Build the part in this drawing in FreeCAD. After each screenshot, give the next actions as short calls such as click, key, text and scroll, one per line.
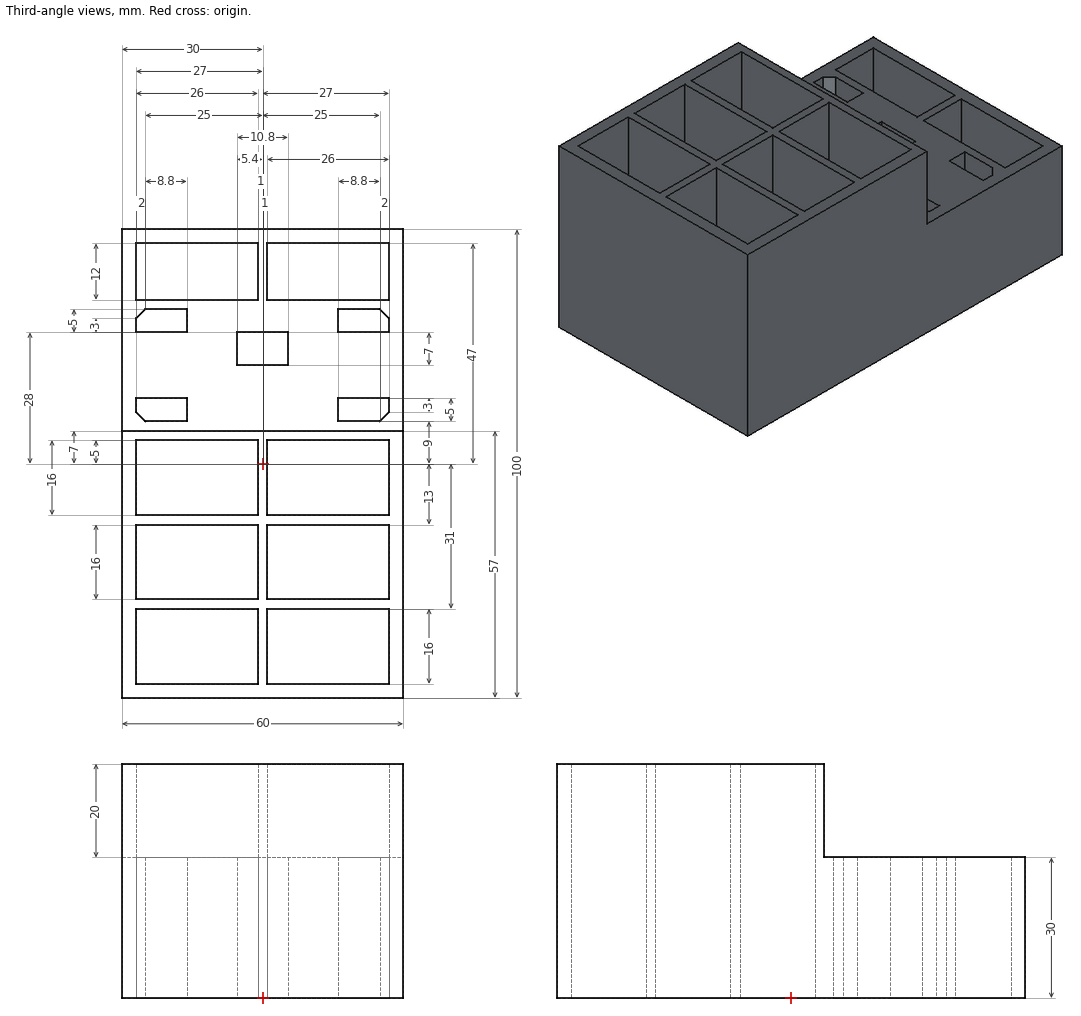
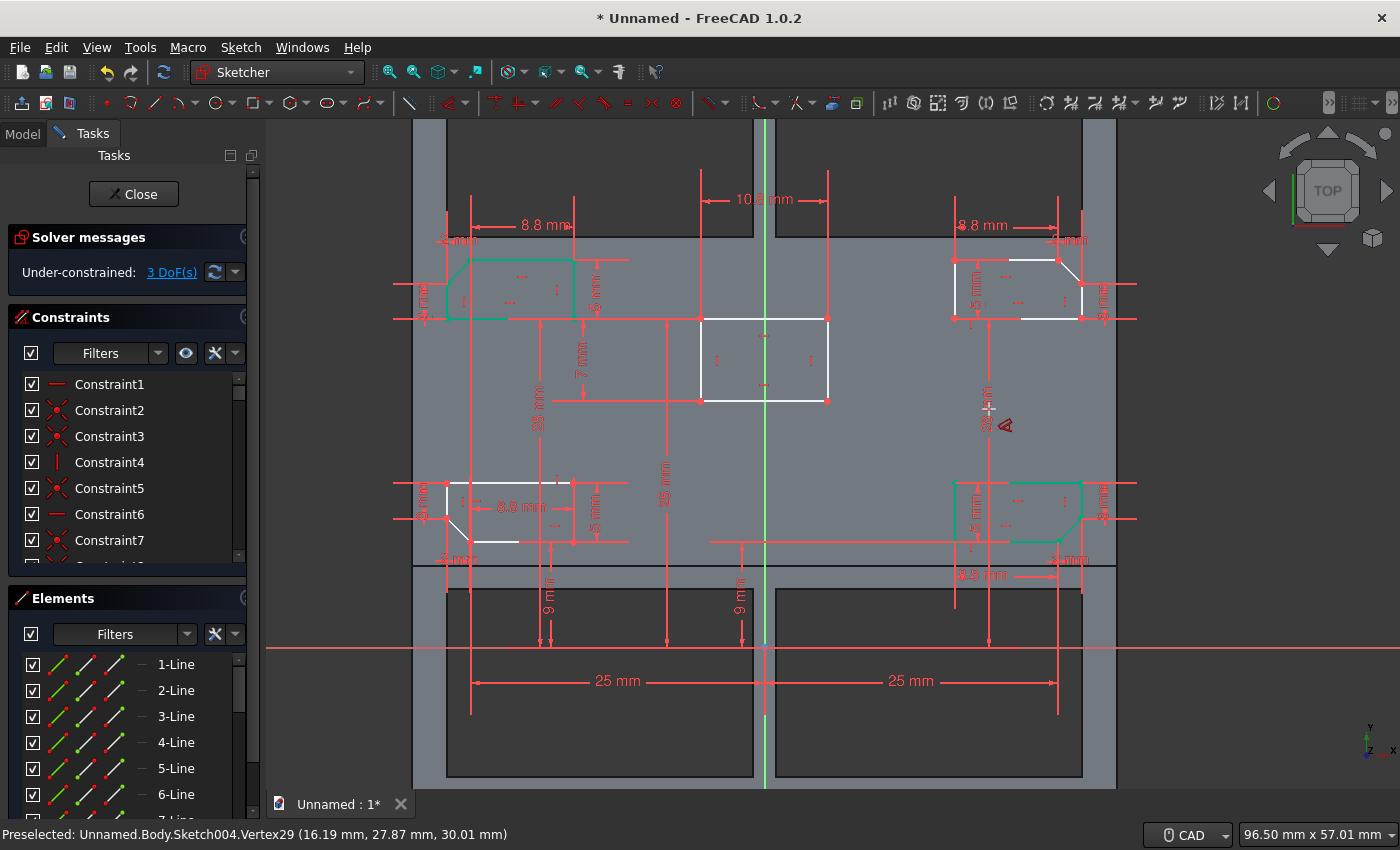
click(1082, 319)
click(996, 682)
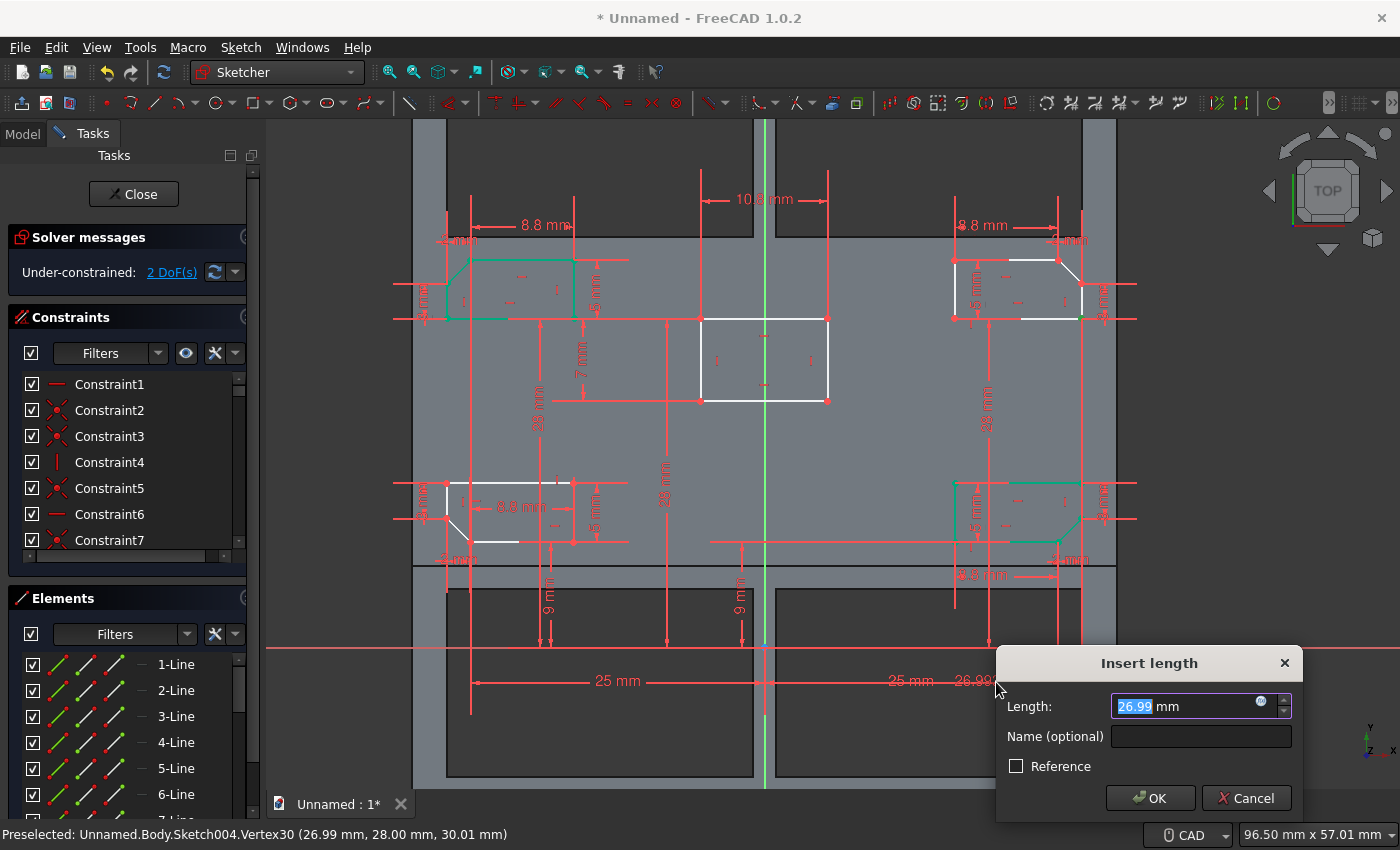
text(27)
key(Return)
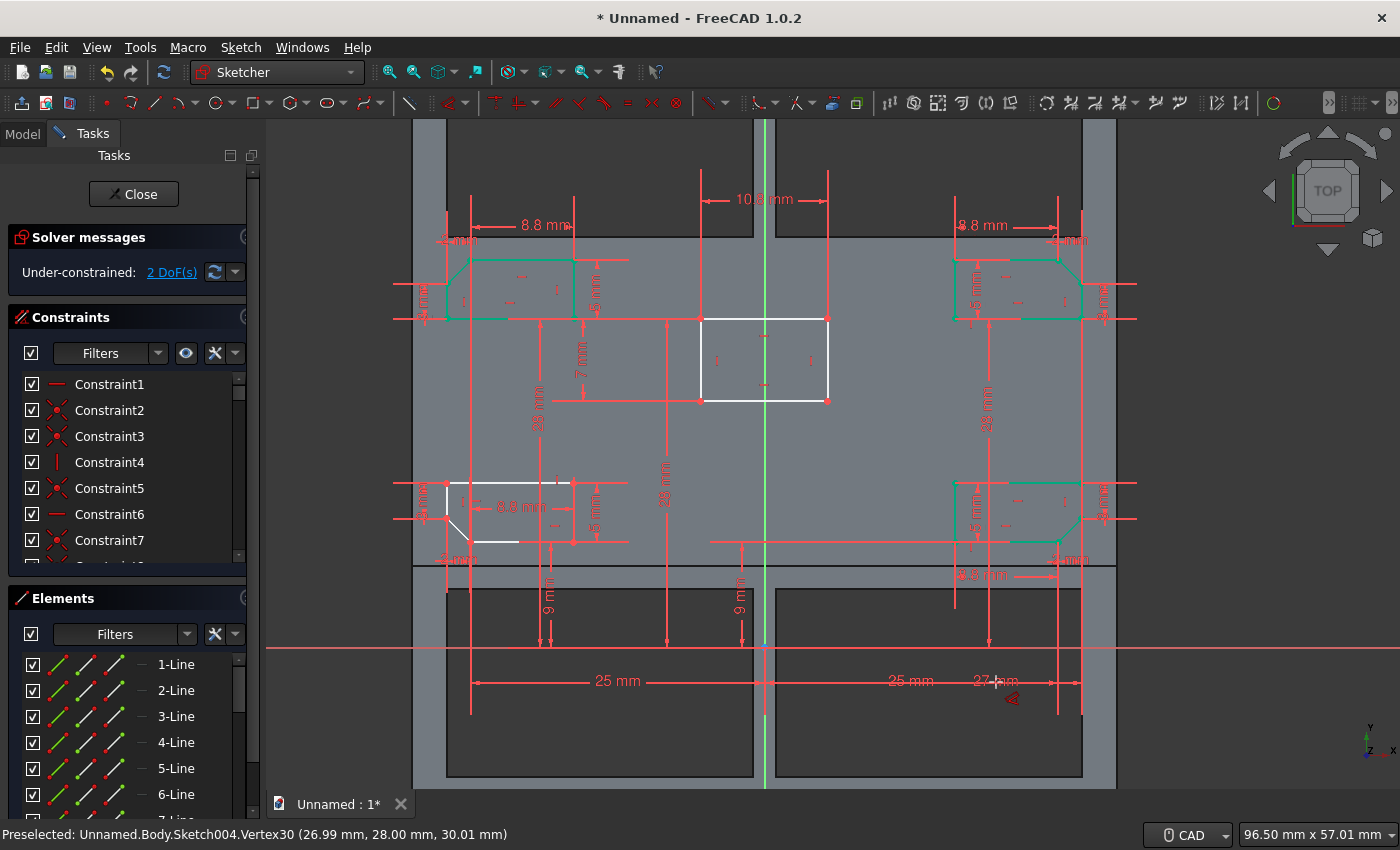
click(447, 483)
click(533, 682)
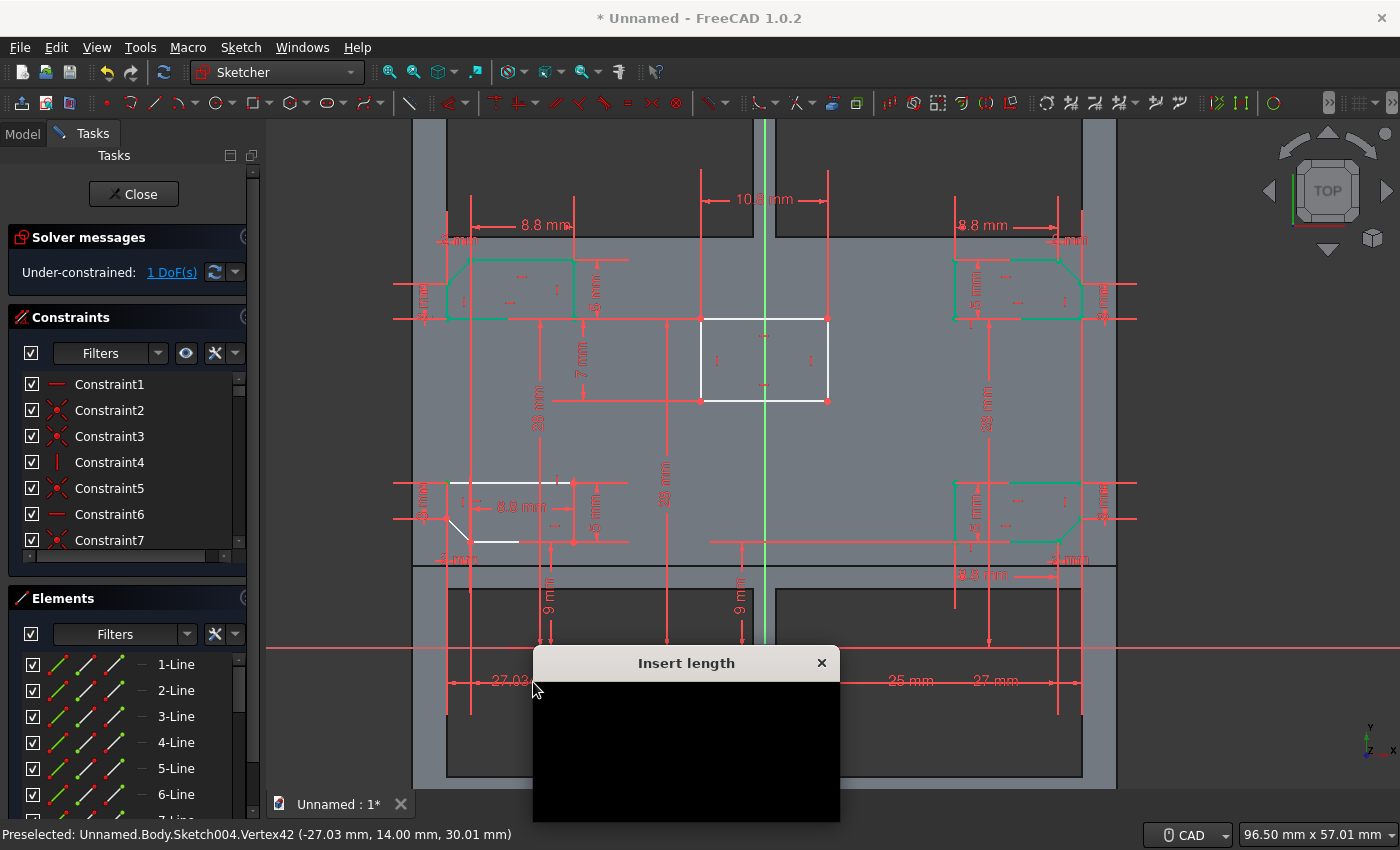
text(27)
key(Return)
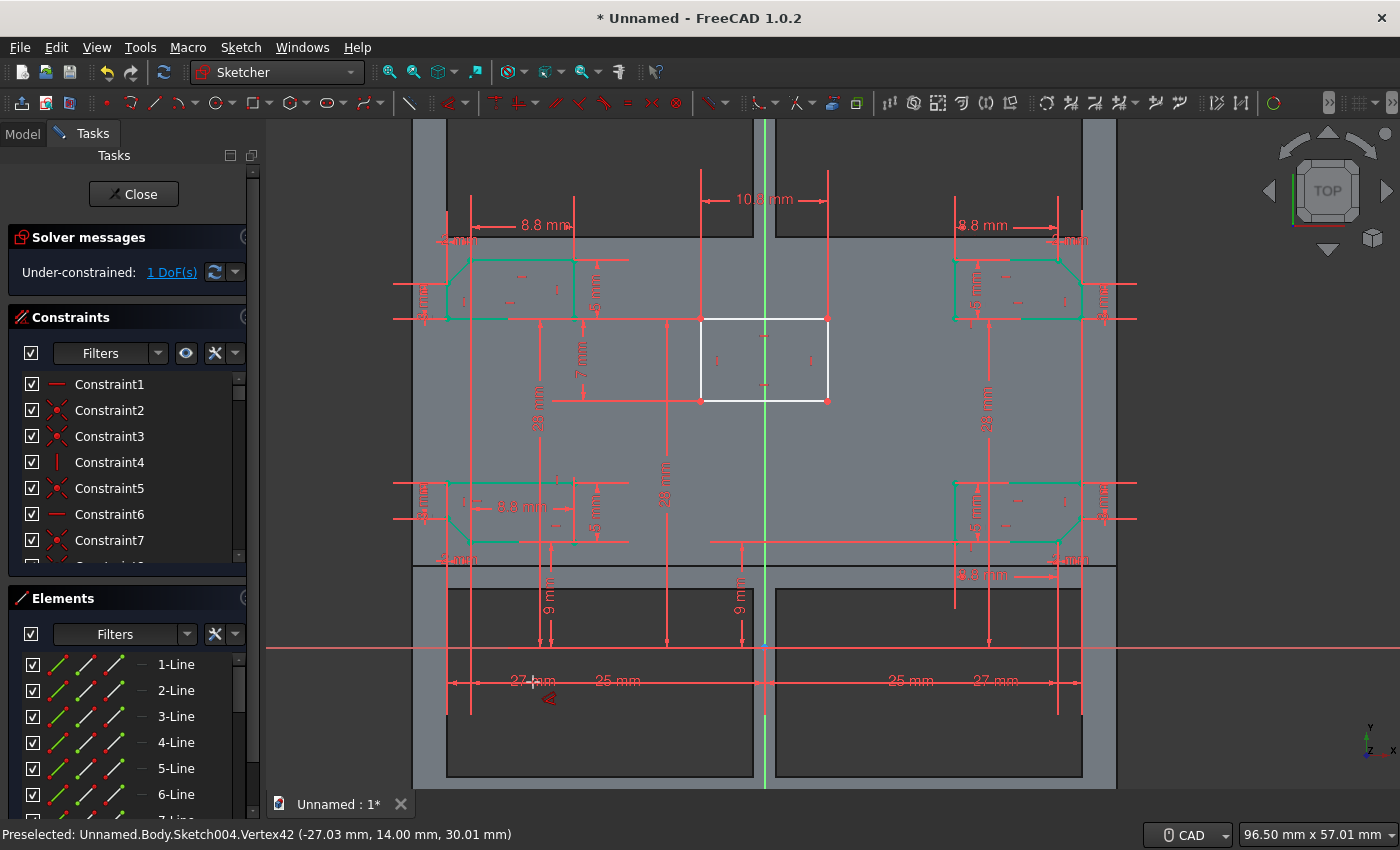
click(701, 319)
click(733, 682)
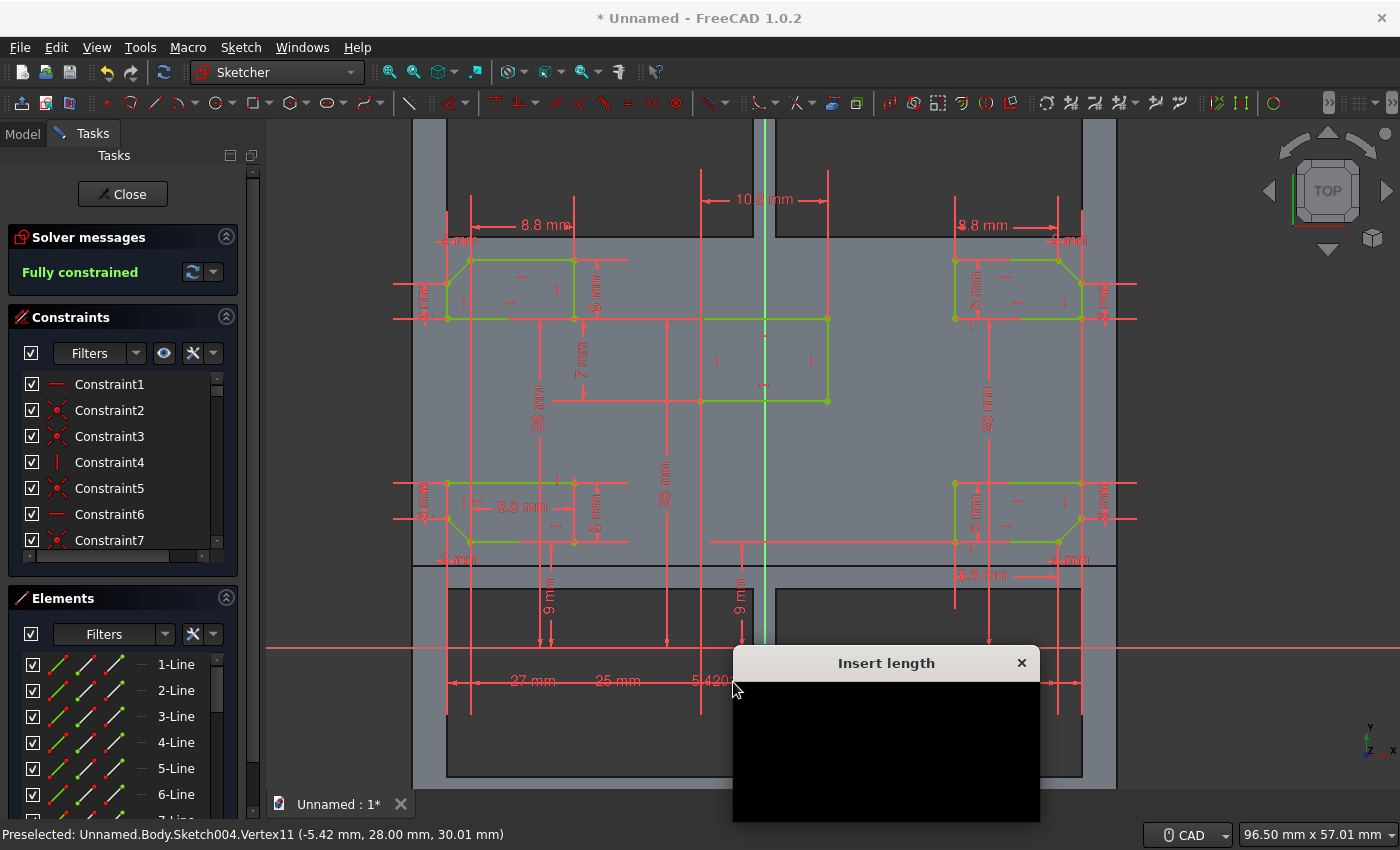
text(5.4)
key(Return)
key(Escape)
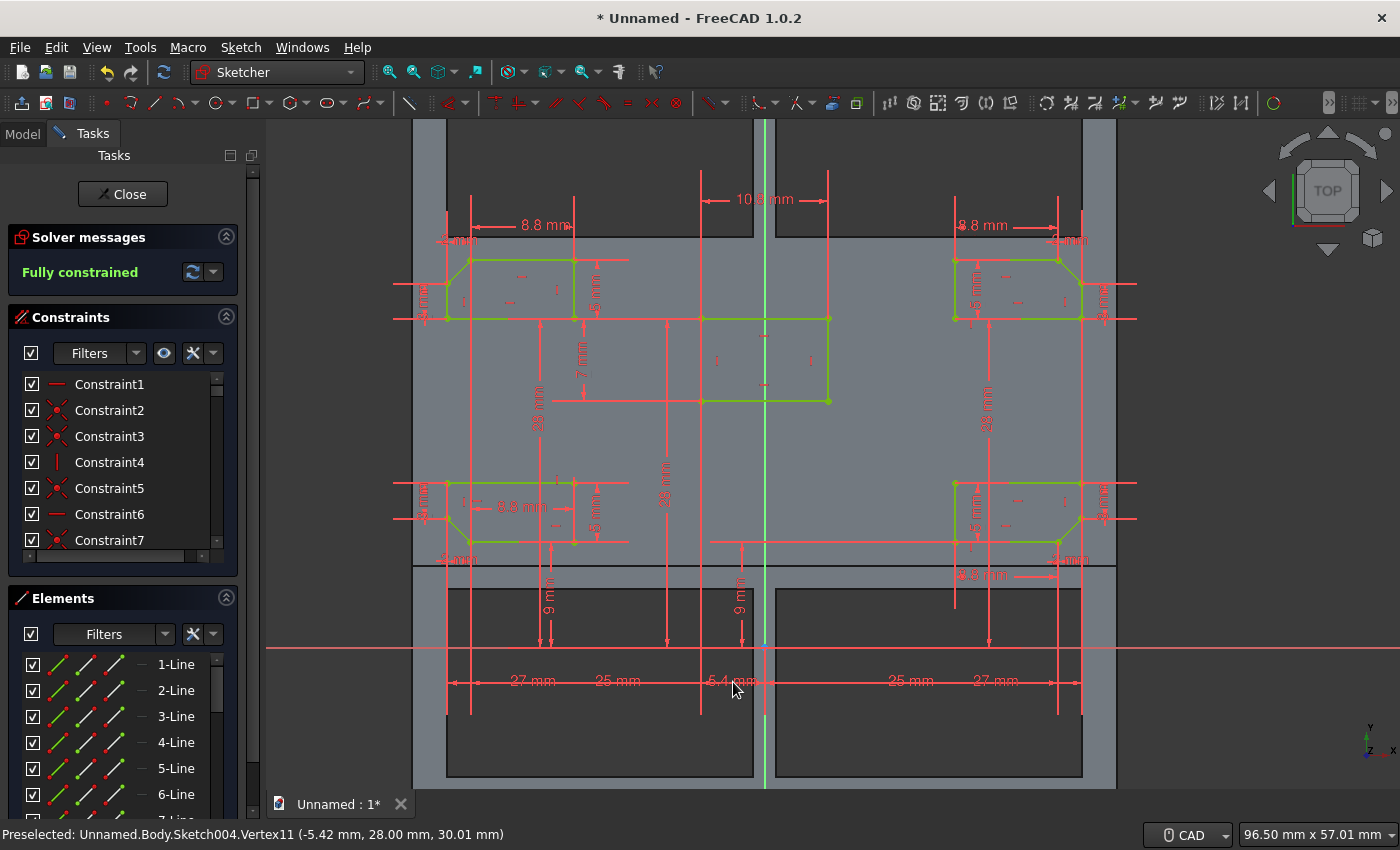
click(123, 194)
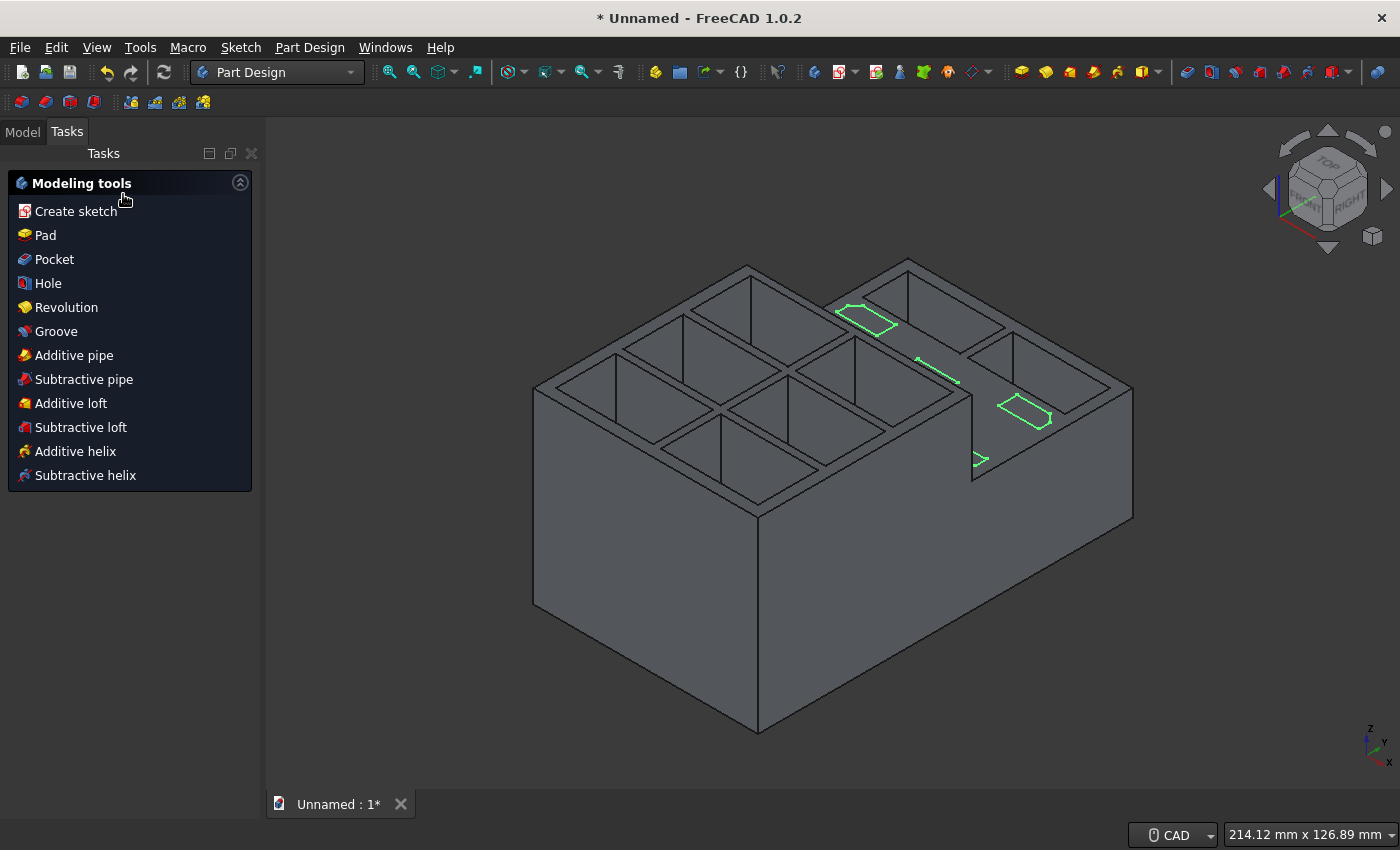
click(1188, 72)